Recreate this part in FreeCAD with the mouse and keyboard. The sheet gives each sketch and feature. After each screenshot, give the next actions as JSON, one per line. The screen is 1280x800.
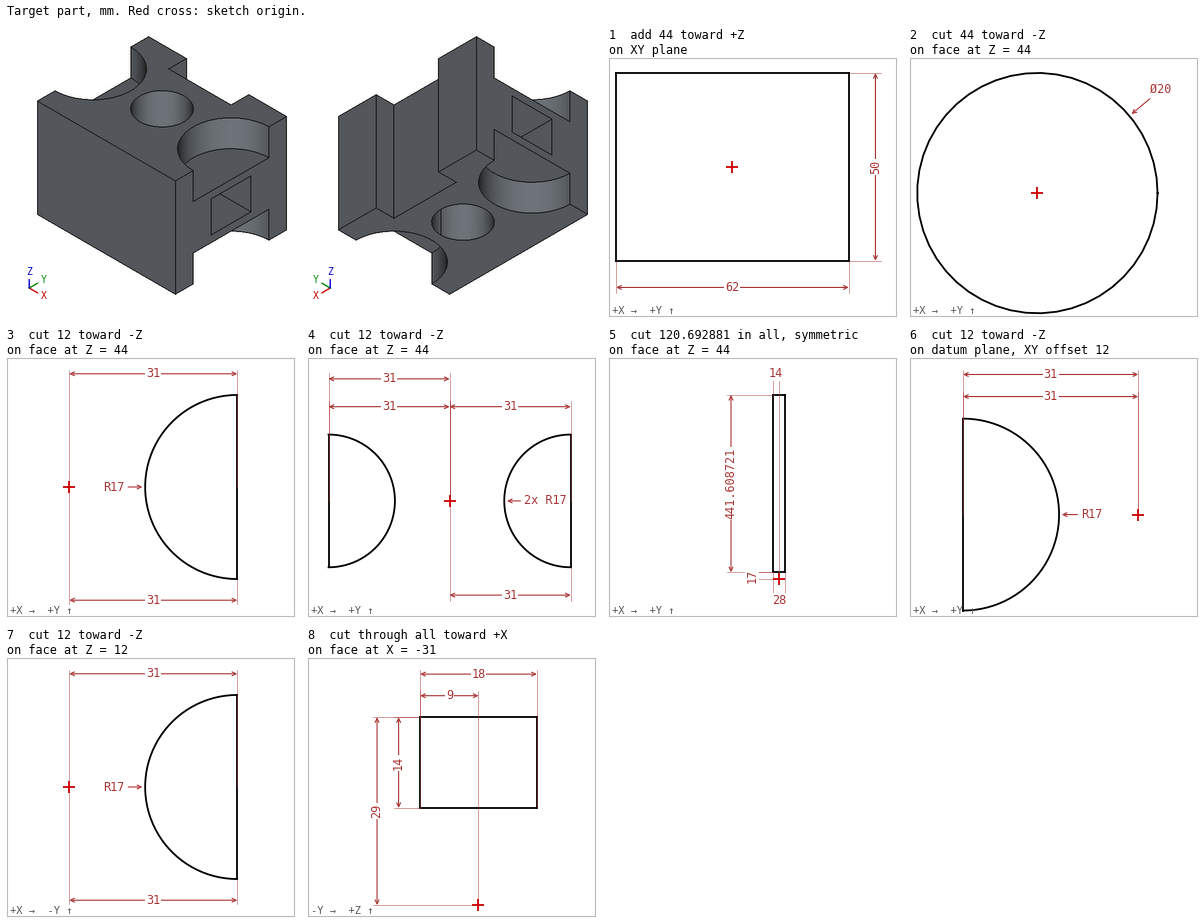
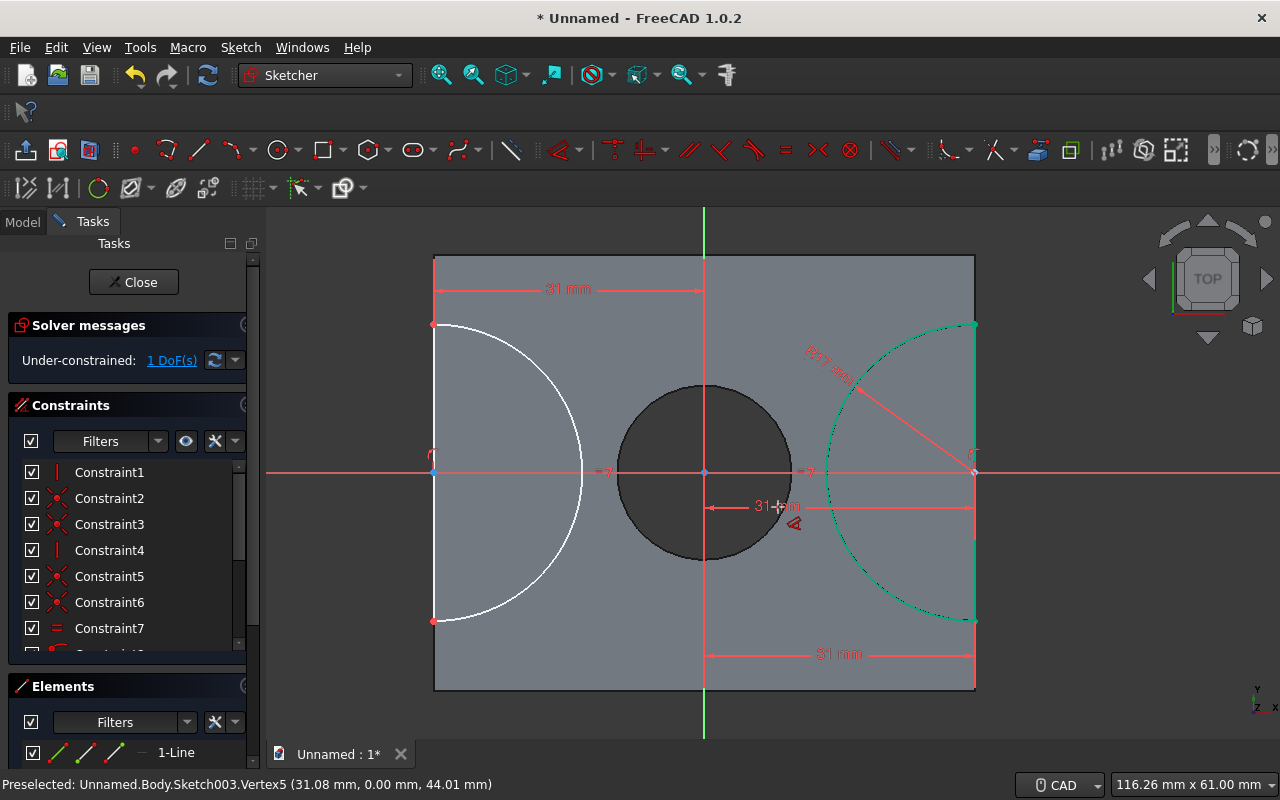
{"action": "left_click", "coordinate": [434, 473]}
{"action": "left_click", "coordinate": [507, 507]}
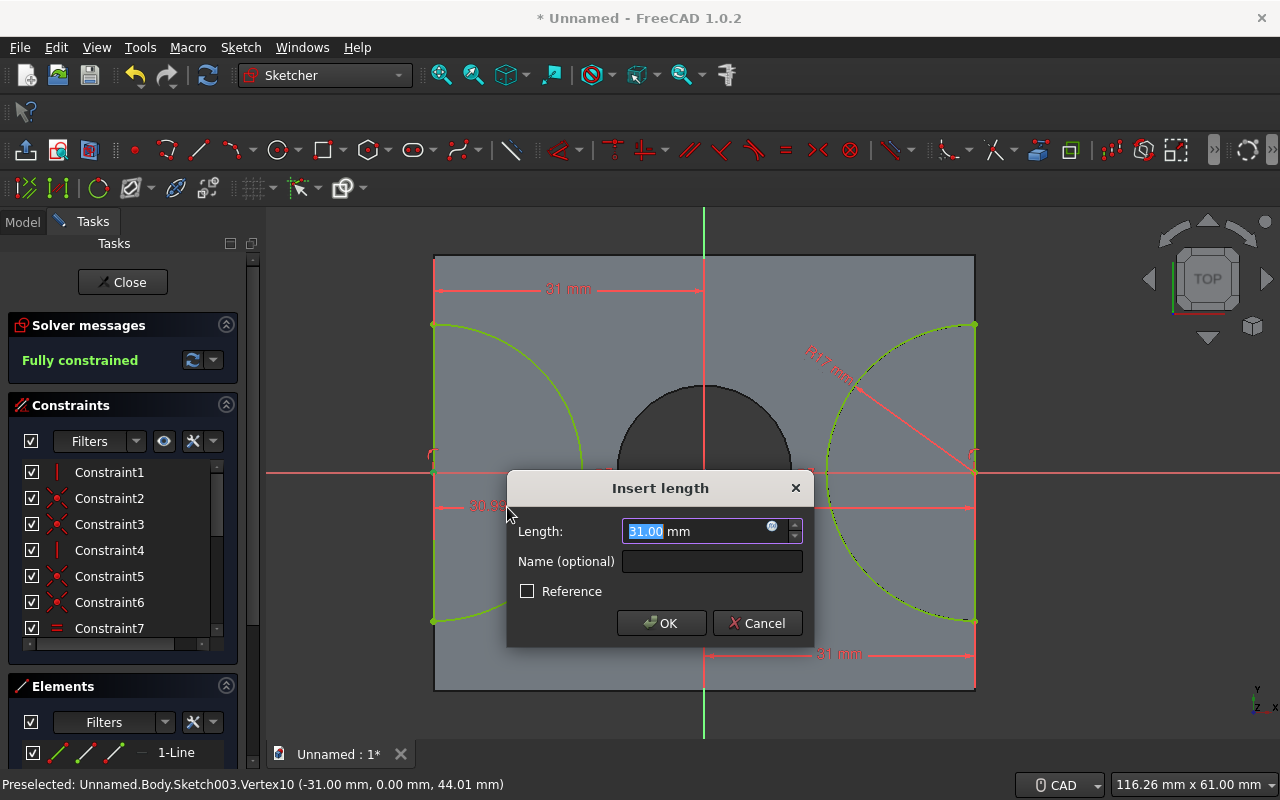
{"action": "type", "text": "31"}
{"action": "key", "text": "Return"}
{"action": "key", "text": "Escape"}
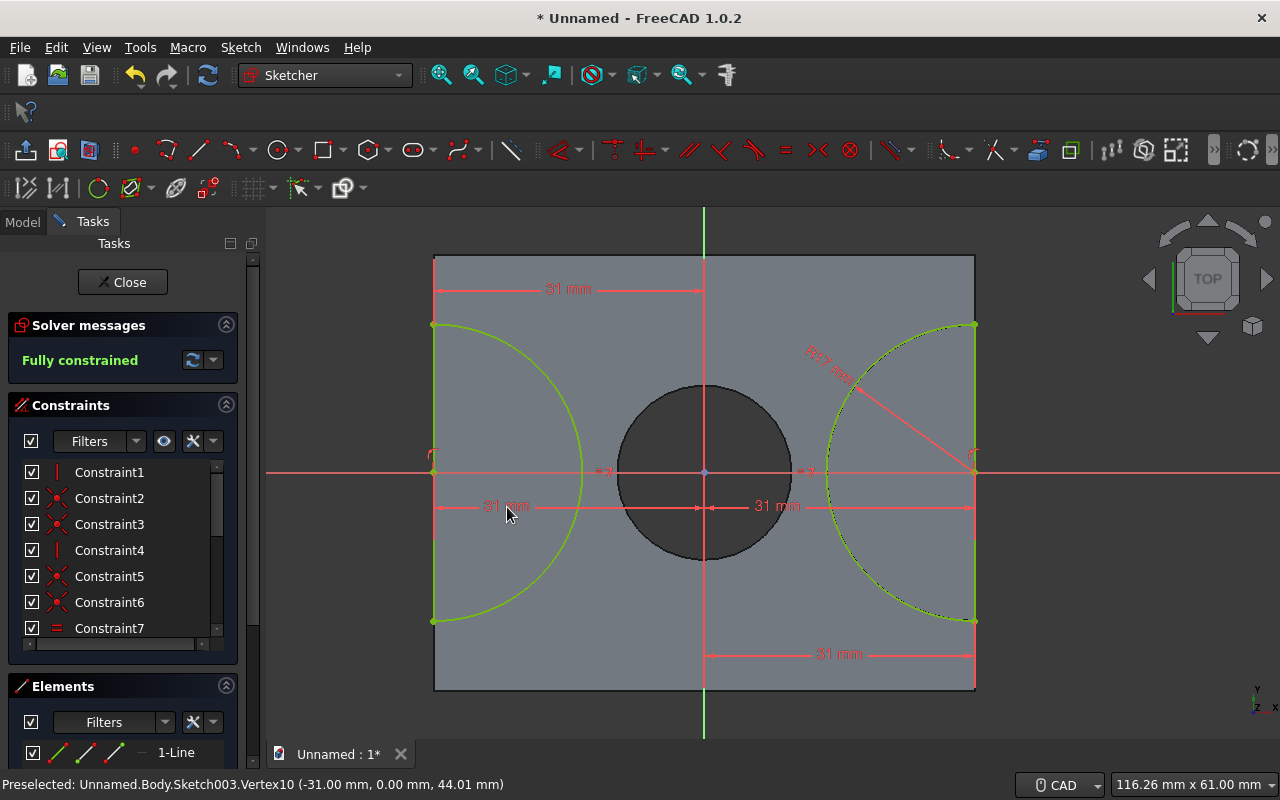
{"action": "left_click", "coordinate": [123, 282]}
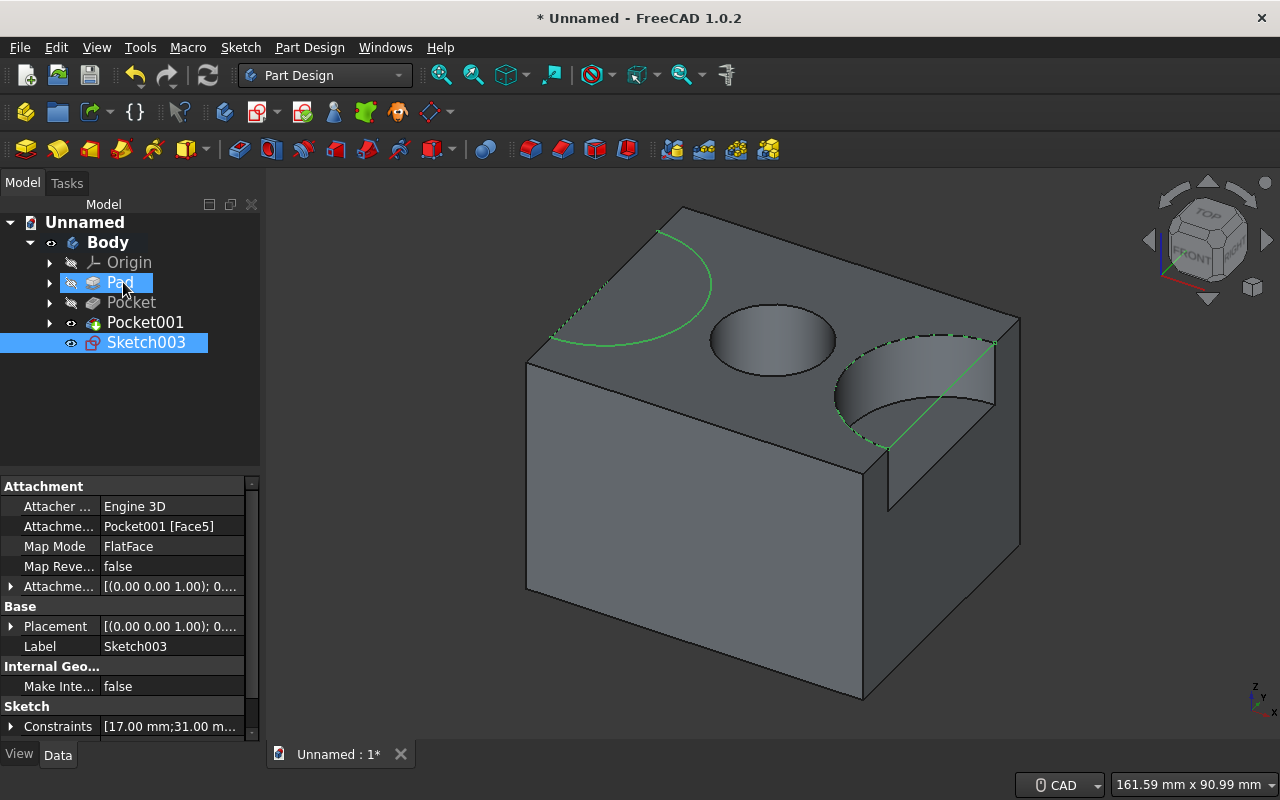
{"action": "left_click", "coordinate": [240, 150]}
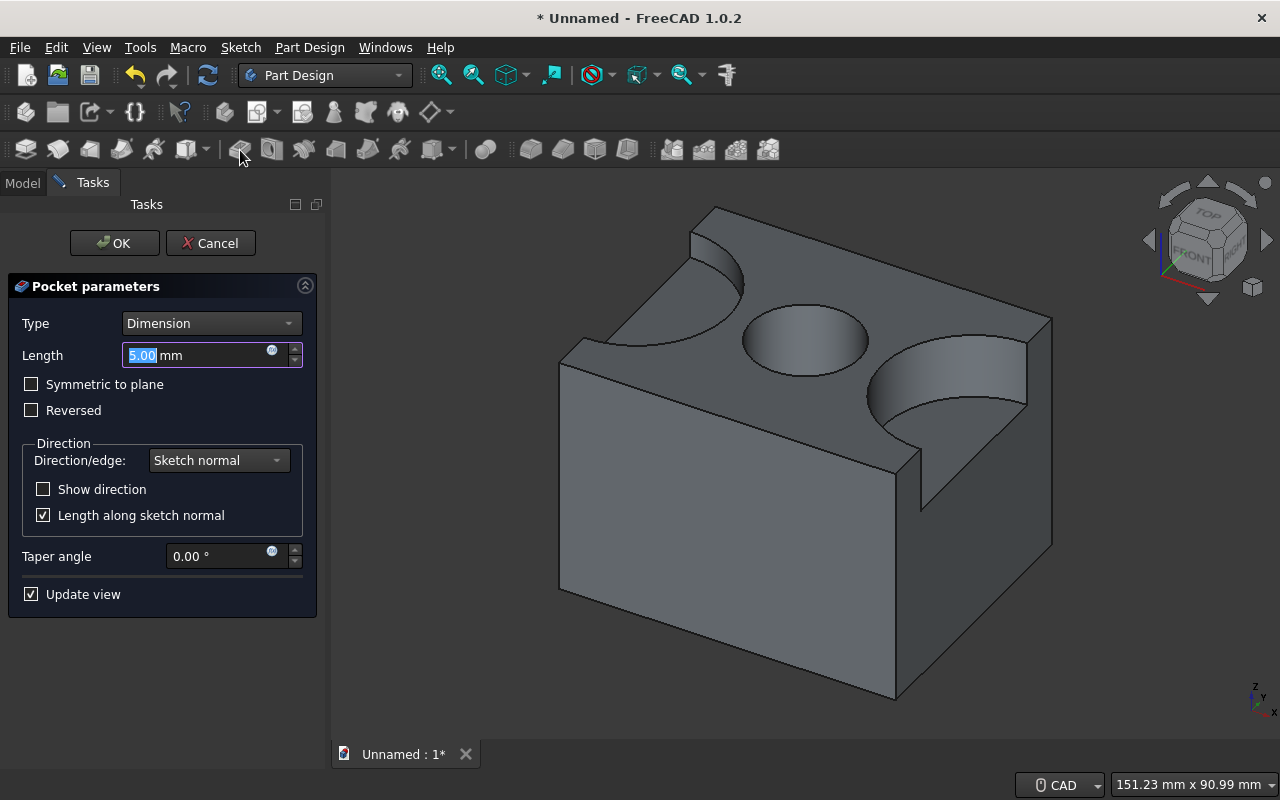
{"action": "type", "text": "12"}
{"action": "key", "text": "Tab"}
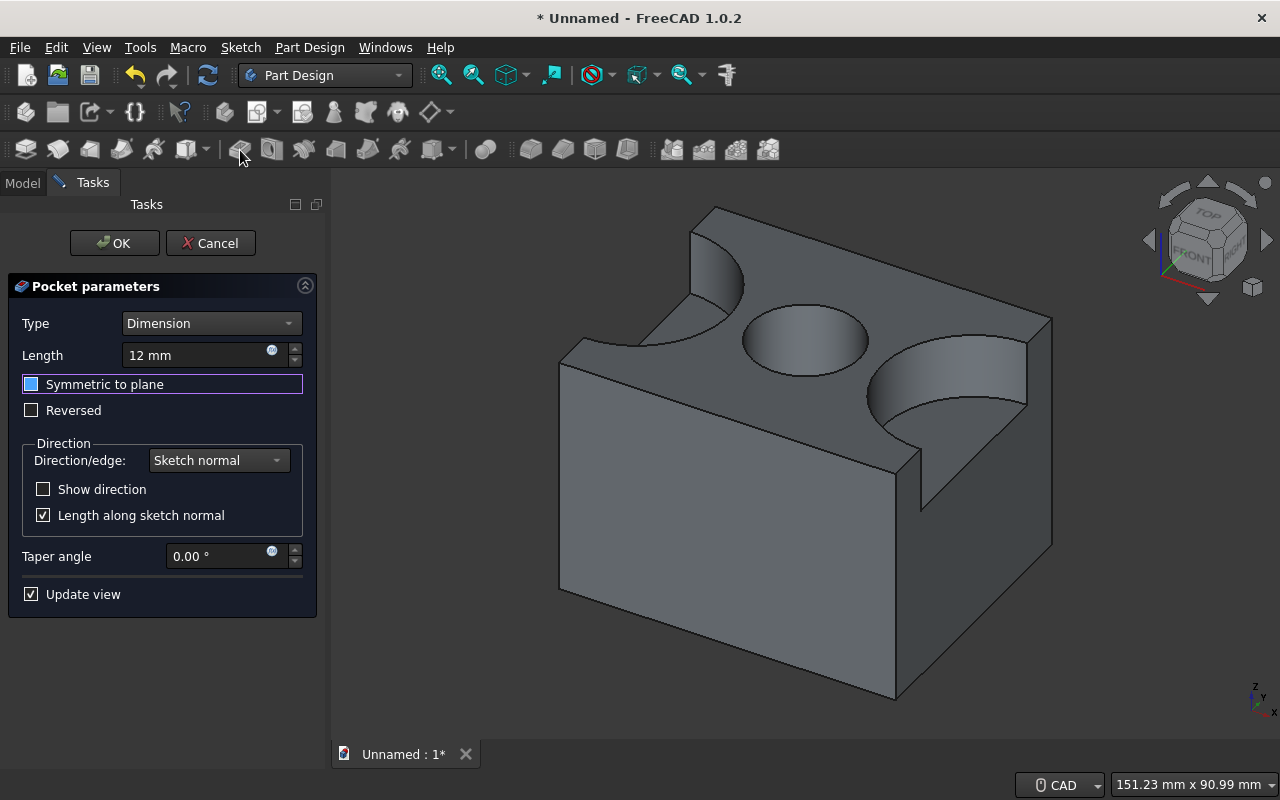
{"action": "left_click", "coordinate": [115, 243]}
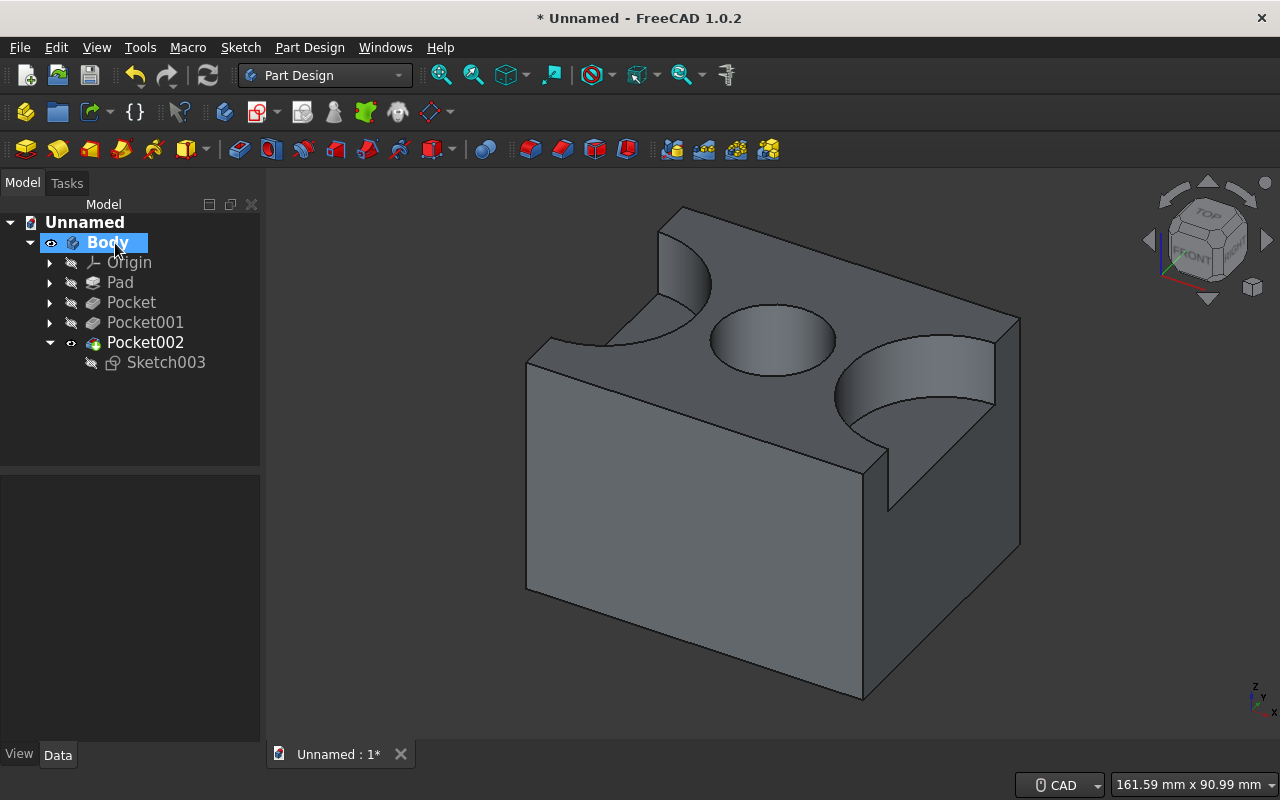
{"action": "left_click", "coordinate": [680, 368]}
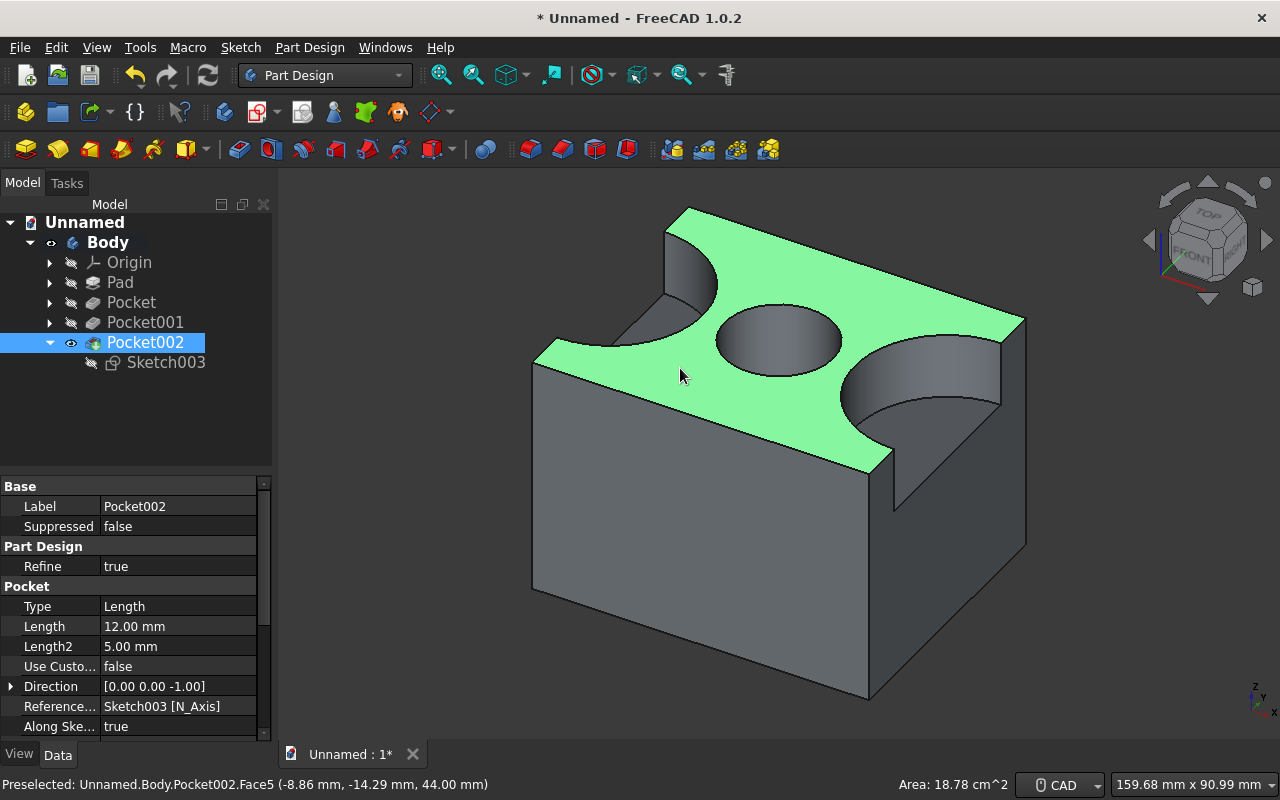
{"action": "left_click", "coordinate": [258, 112]}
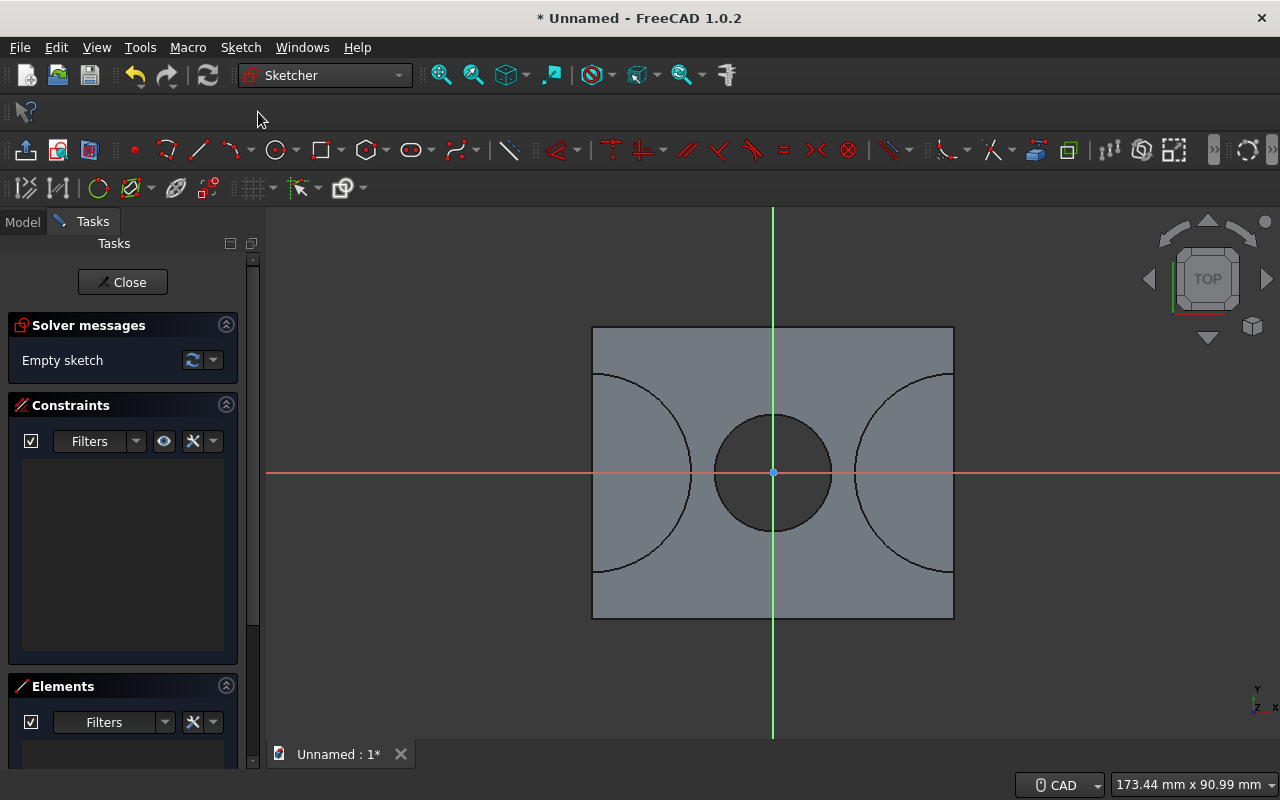
{"action": "scroll", "coordinate": [694, 683], "scroll_direction": "down", "scroll_amount": 10}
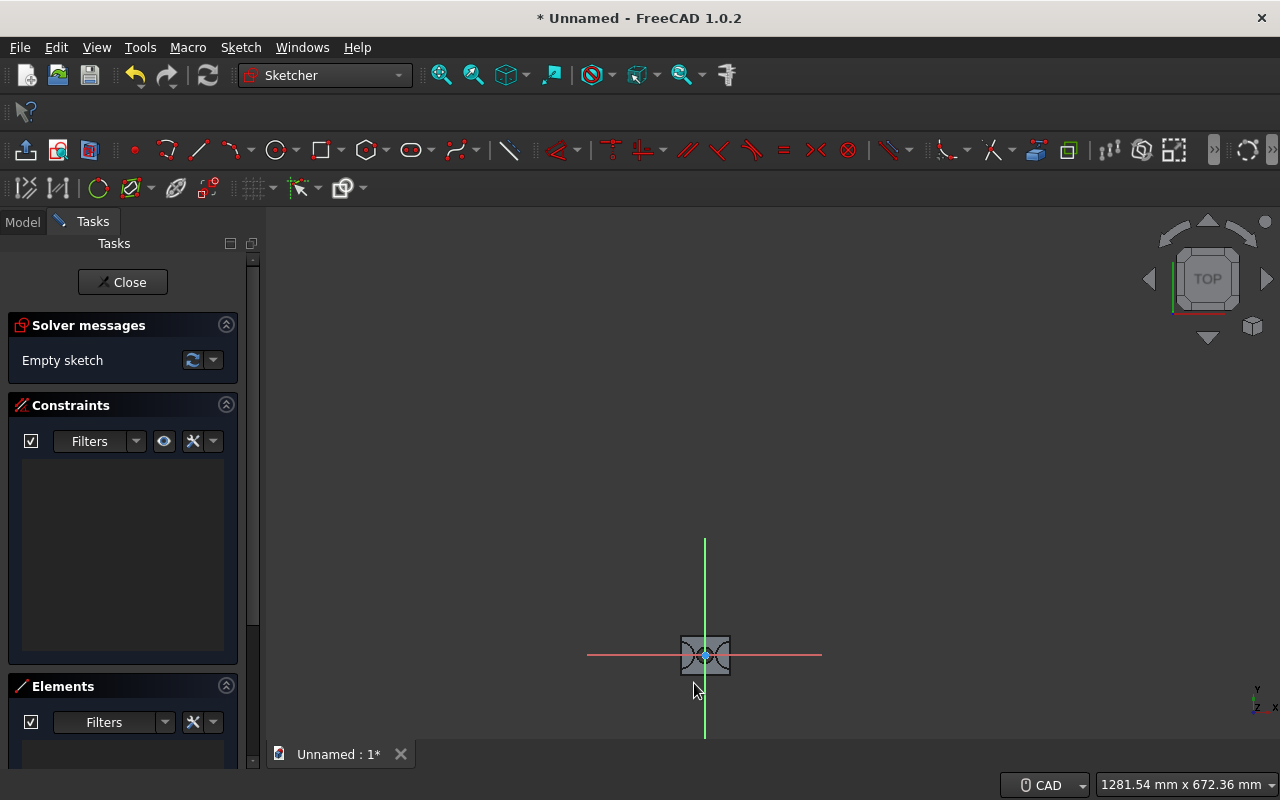
{"action": "key", "text": "g r"}